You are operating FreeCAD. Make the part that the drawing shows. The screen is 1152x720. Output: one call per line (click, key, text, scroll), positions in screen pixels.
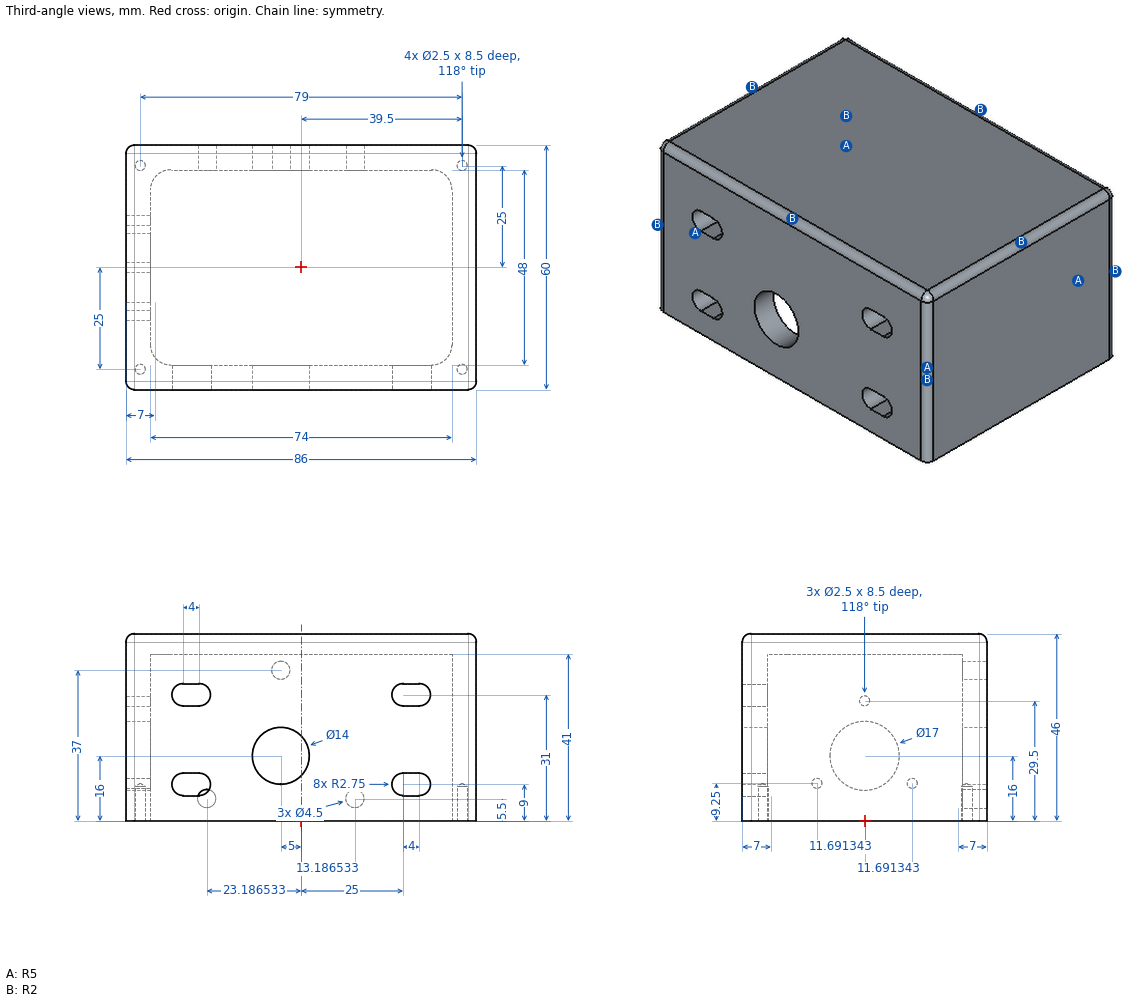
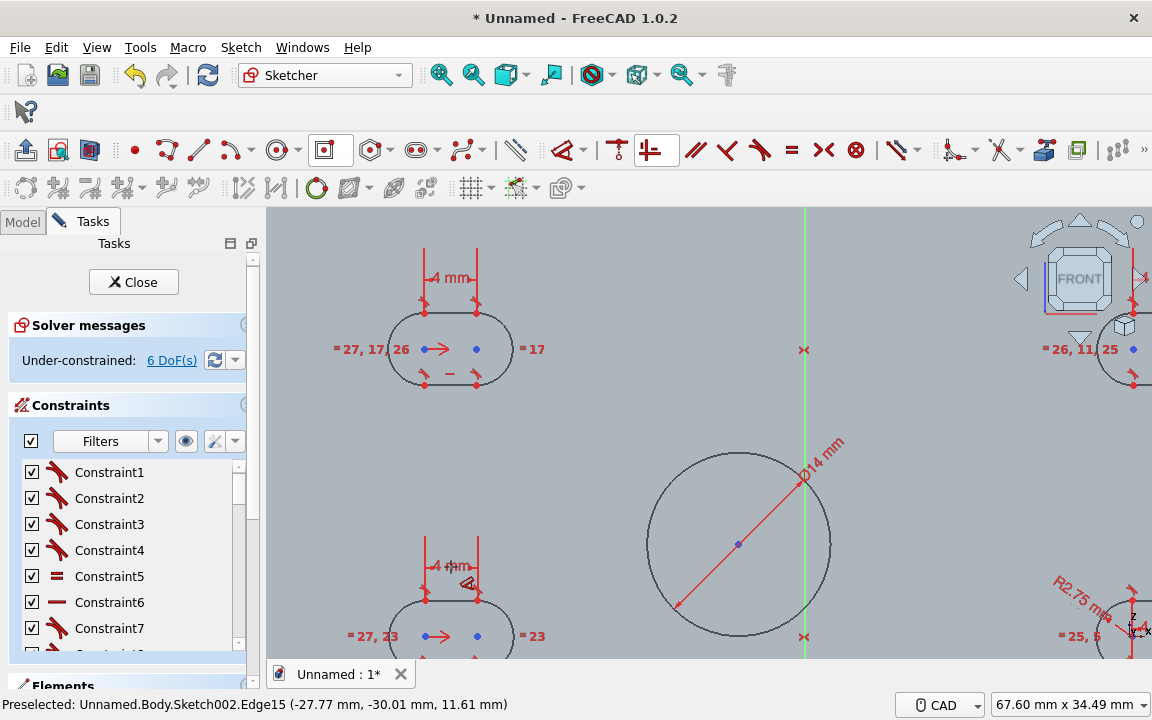
click(739, 544)
click(772, 510)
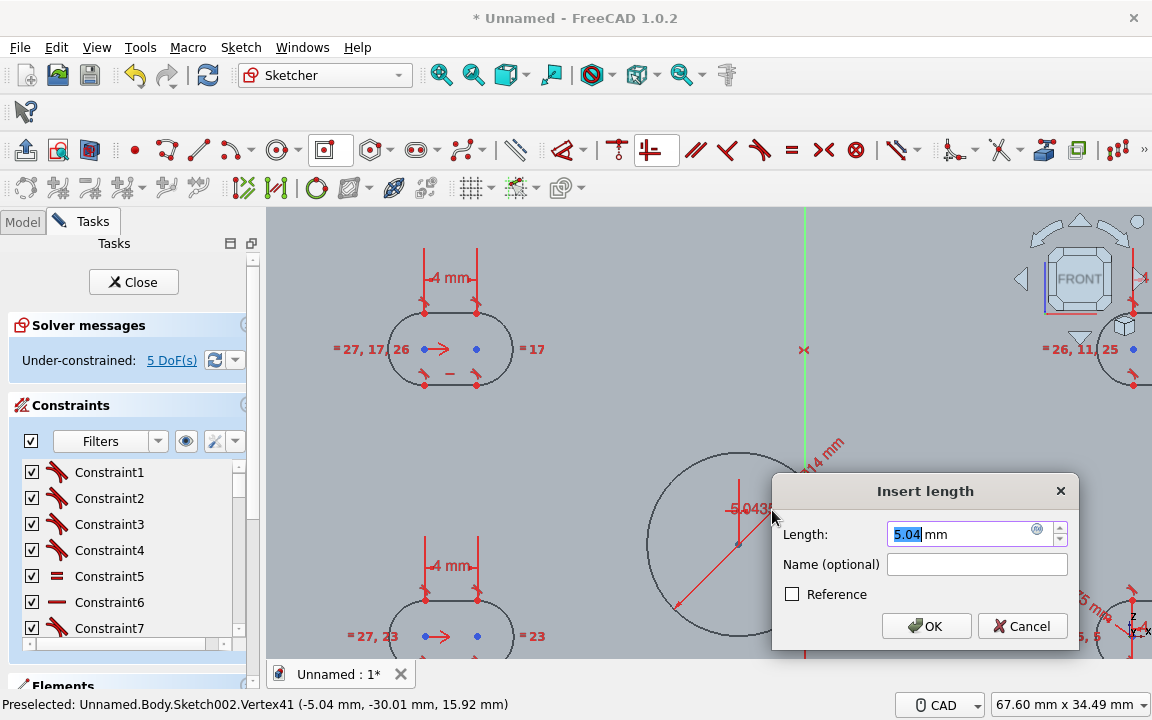
text(5)
key(Return)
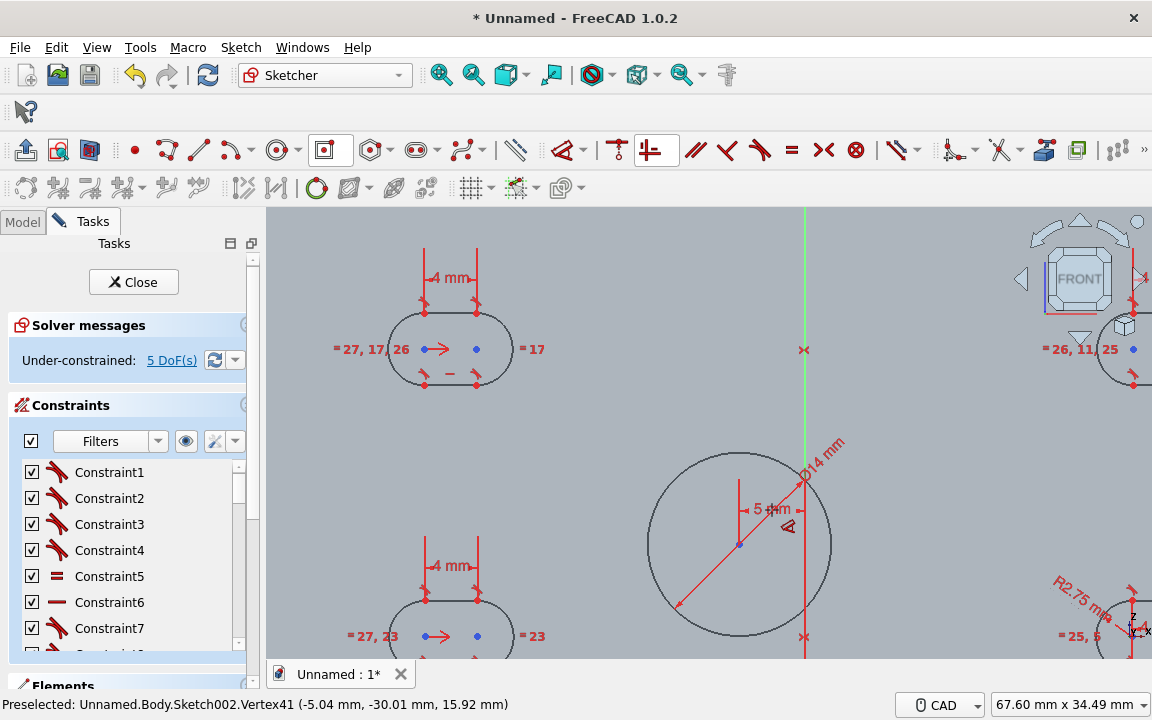
scroll(440, 313, down, 3)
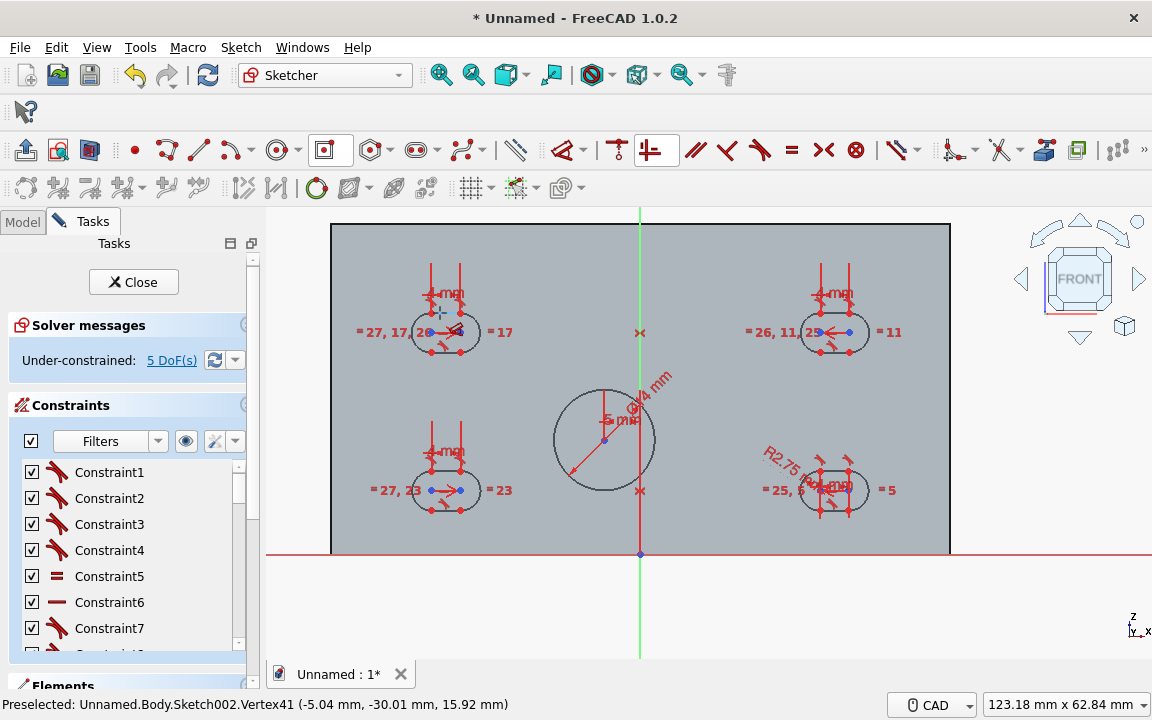
click(820, 491)
click(854, 537)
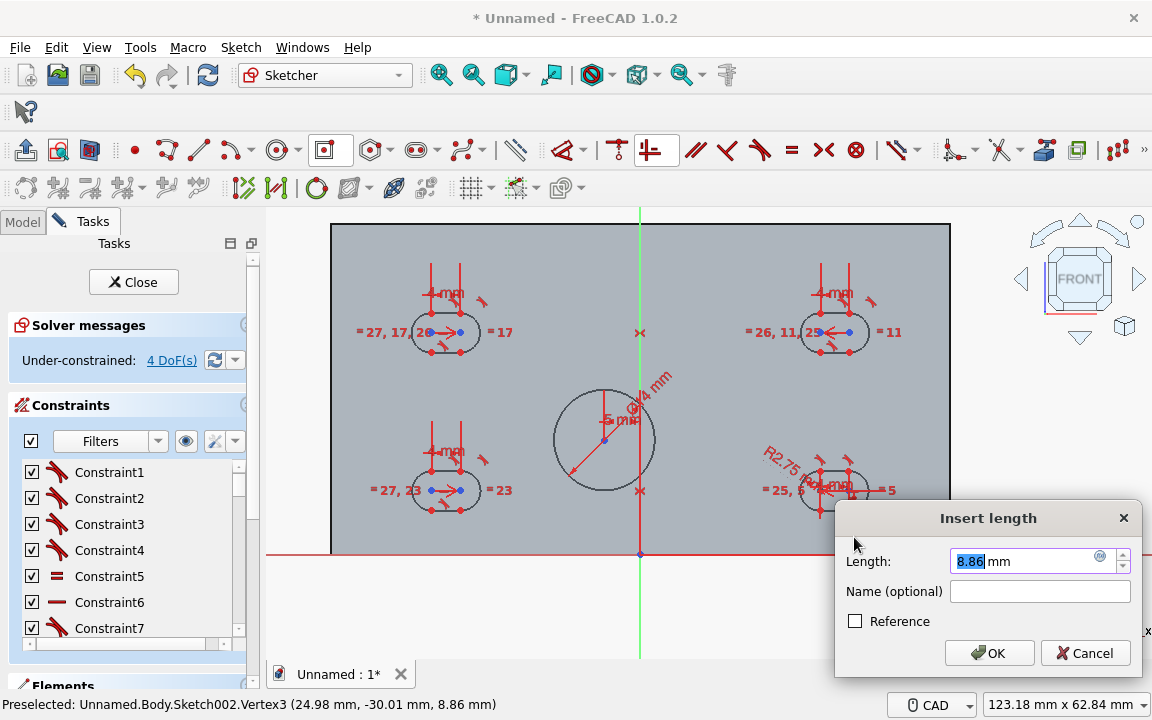
text(9)
key(Return)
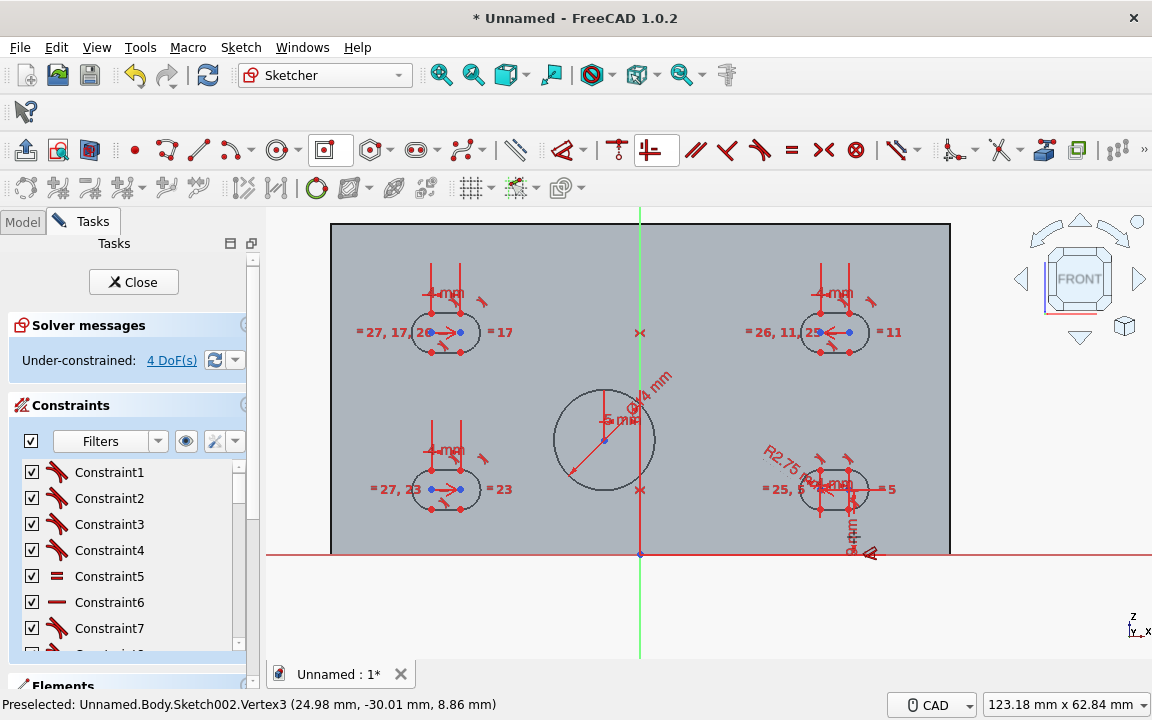
click(604, 440)
click(570, 497)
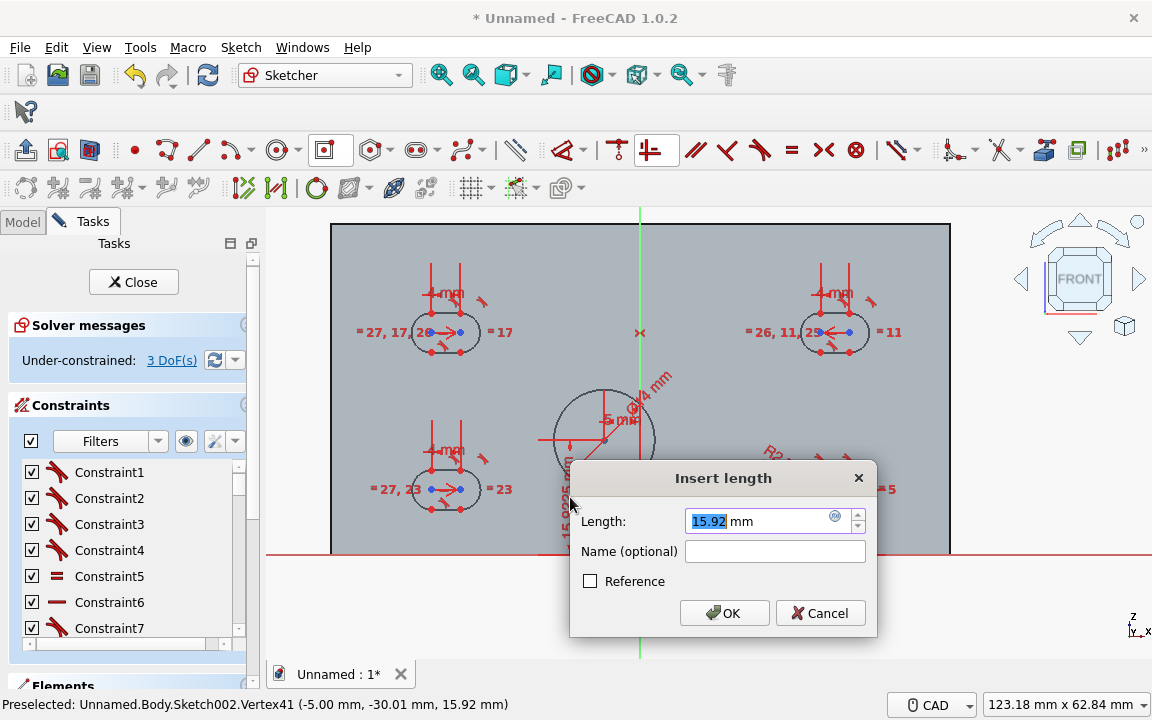
text(16)
key(Return)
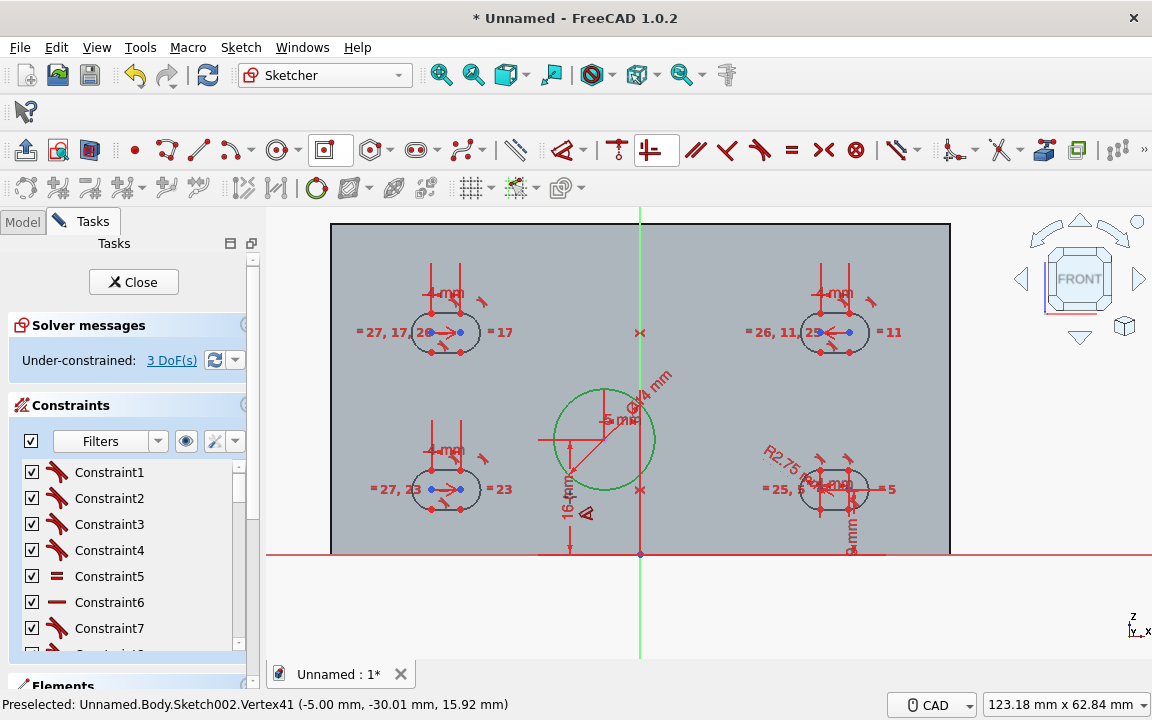
click(820, 470)
click(730, 589)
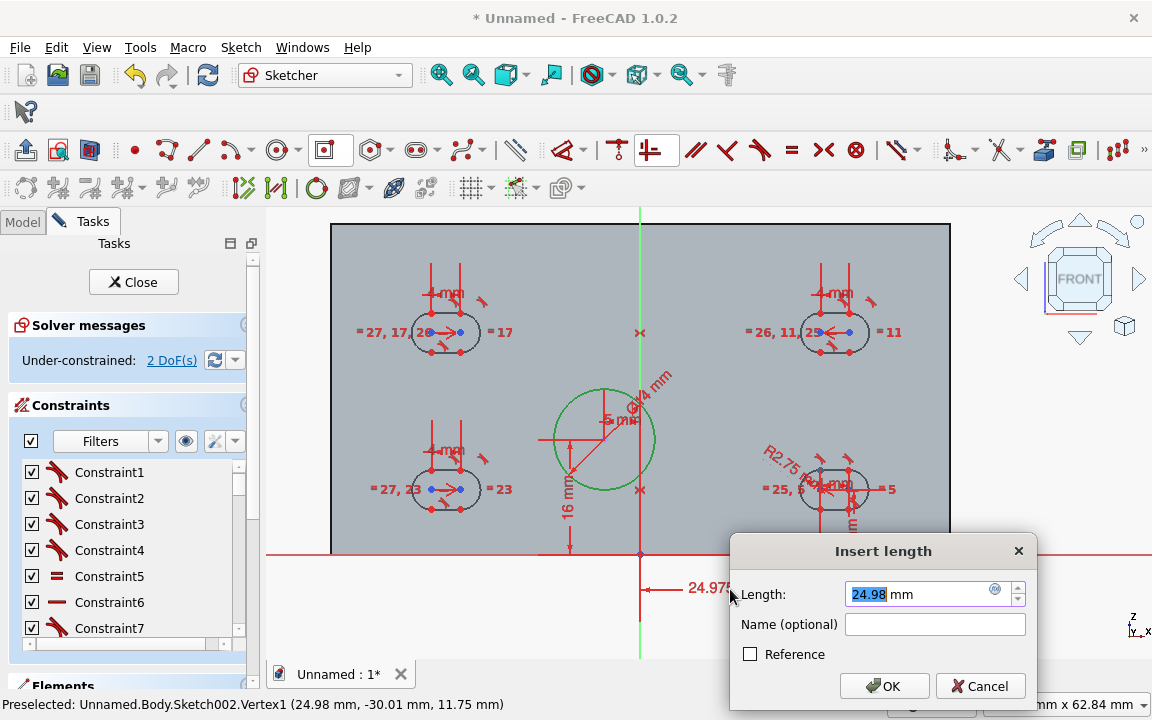
text(25)
key(Return)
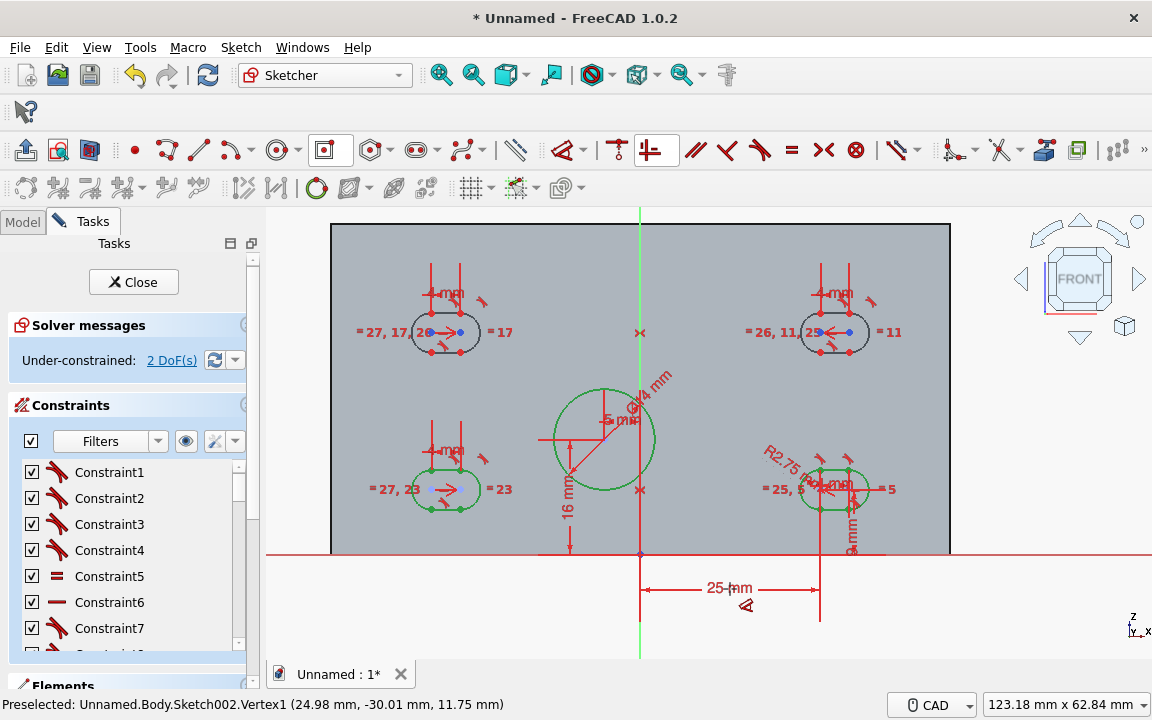
click(821, 313)
click(730, 279)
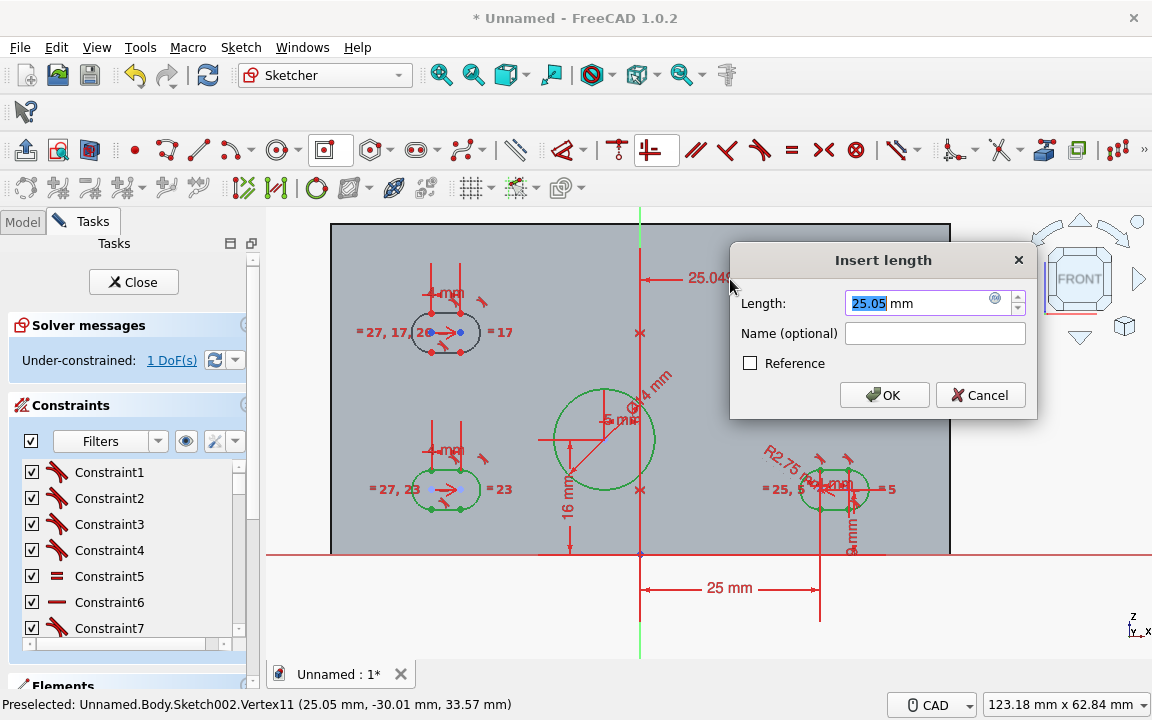
text(25)
key(Return)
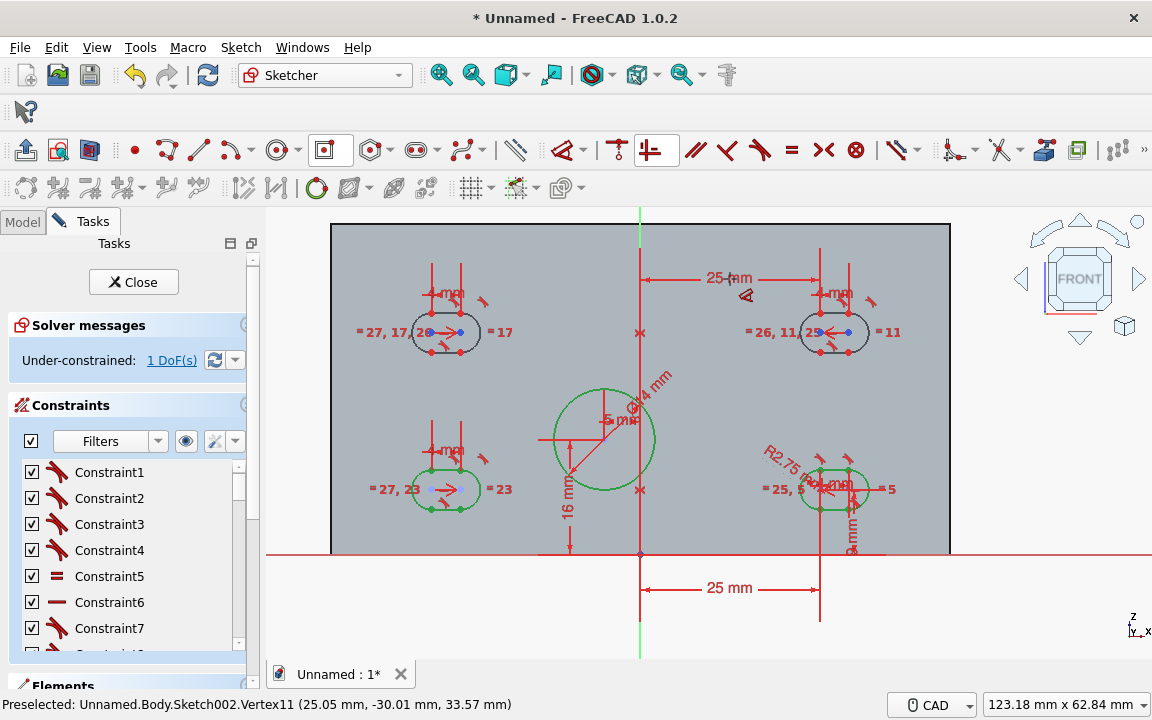
click(820, 333)
click(854, 444)